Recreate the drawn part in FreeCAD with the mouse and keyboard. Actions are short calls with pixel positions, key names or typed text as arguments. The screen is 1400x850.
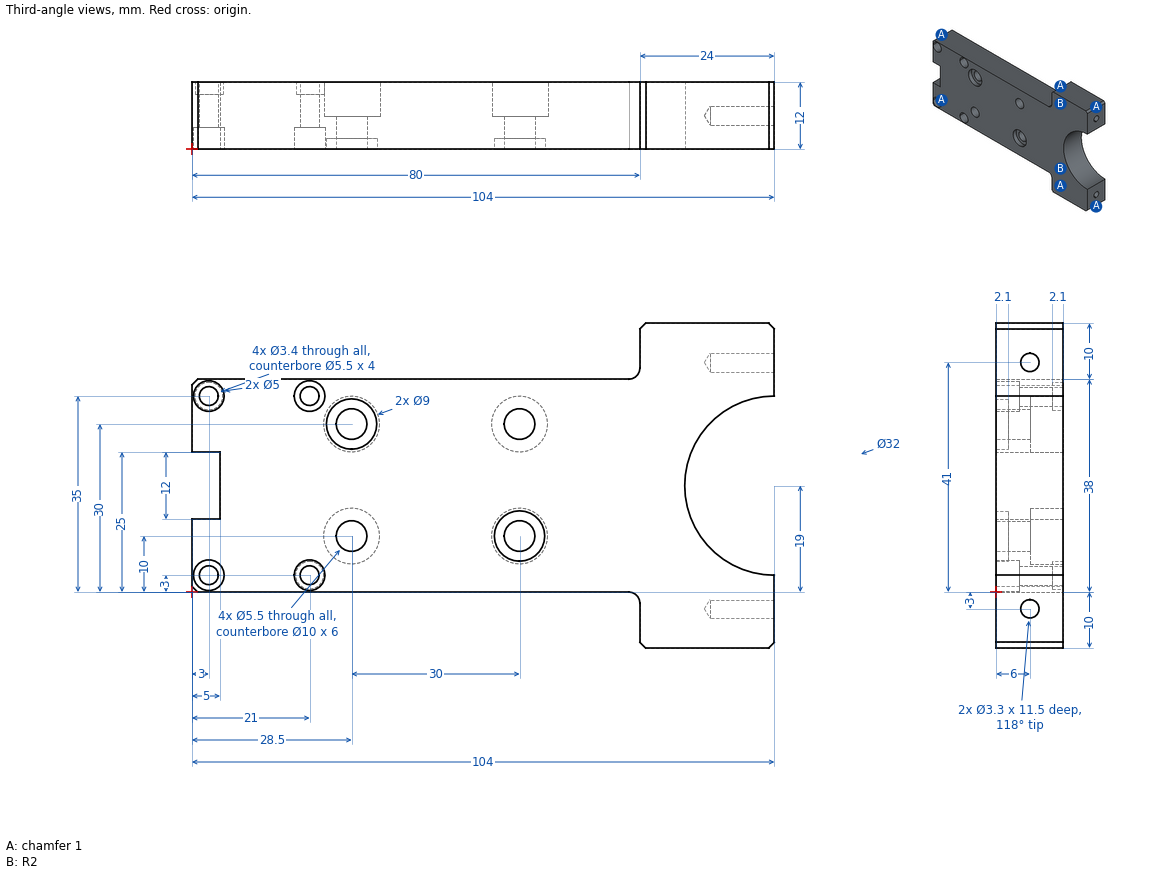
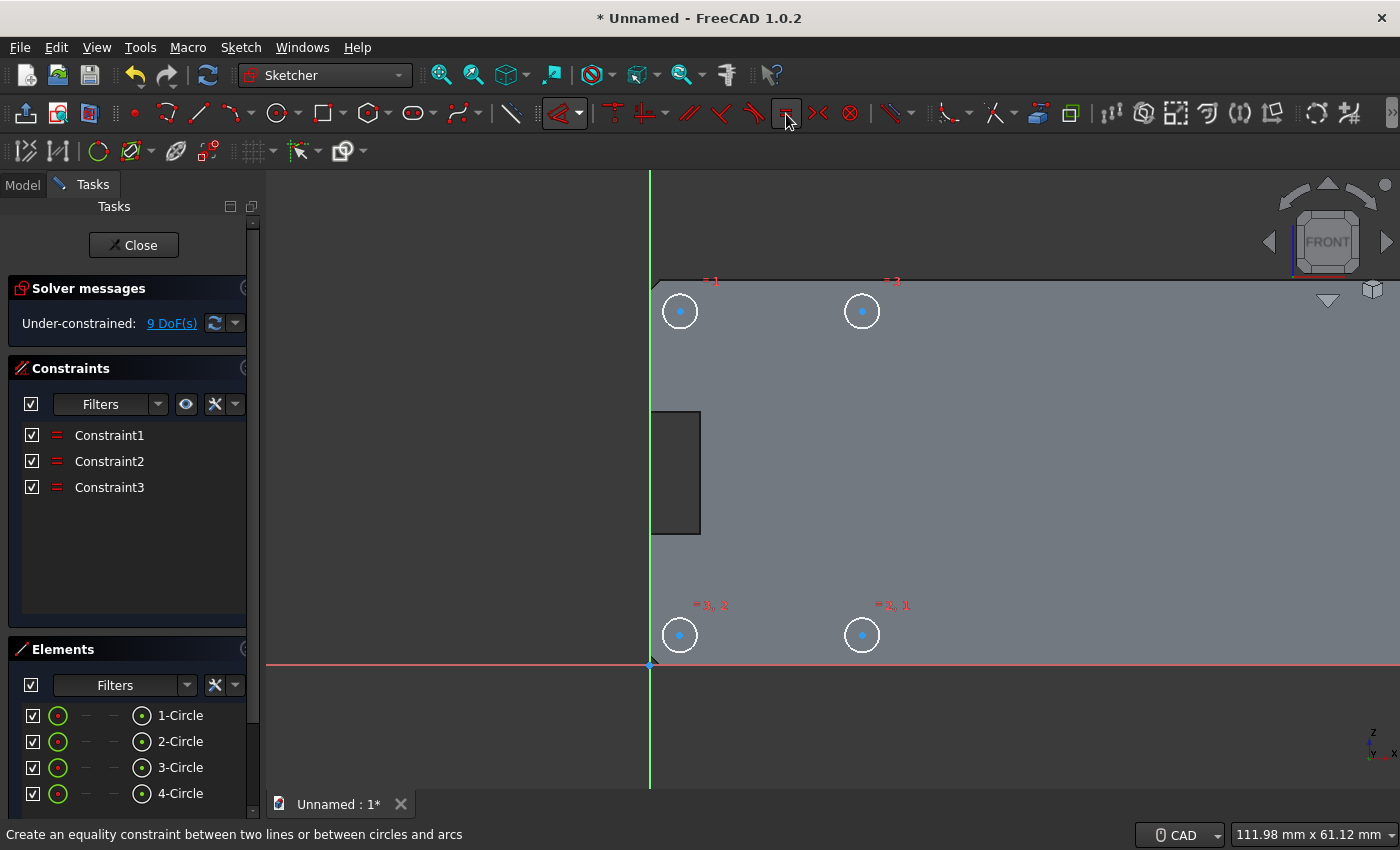
click(680, 311)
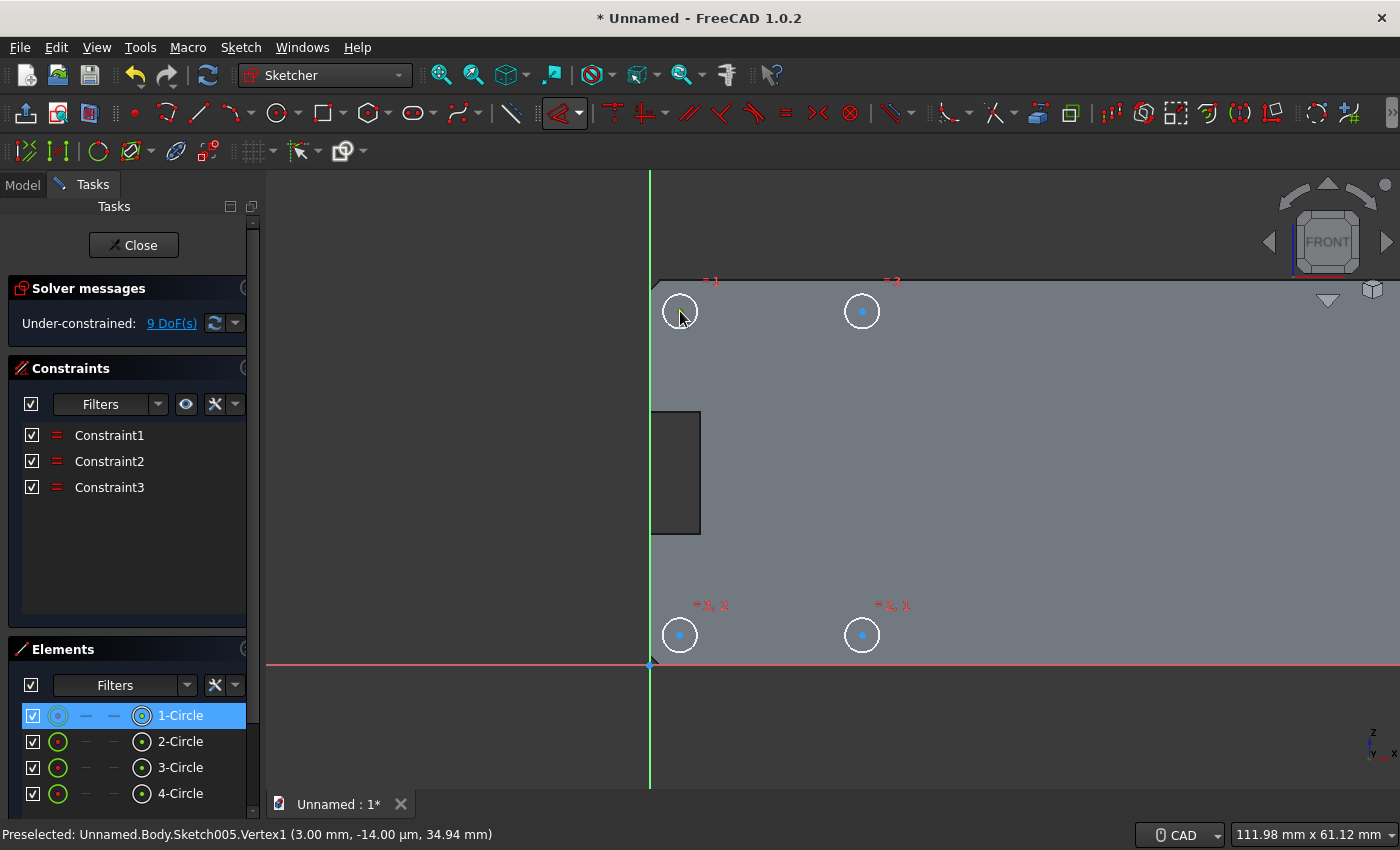
click(680, 635)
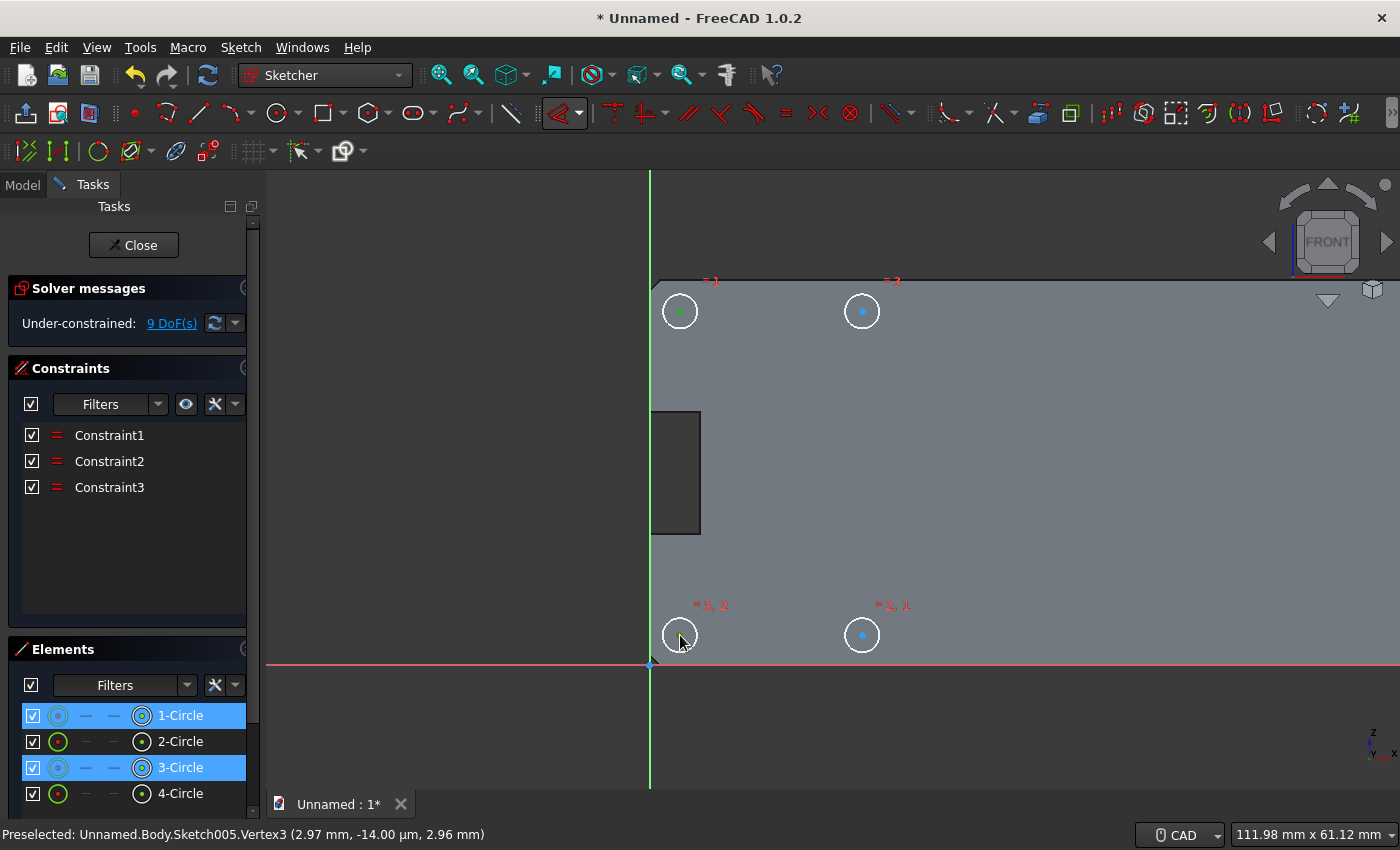
click(668, 114)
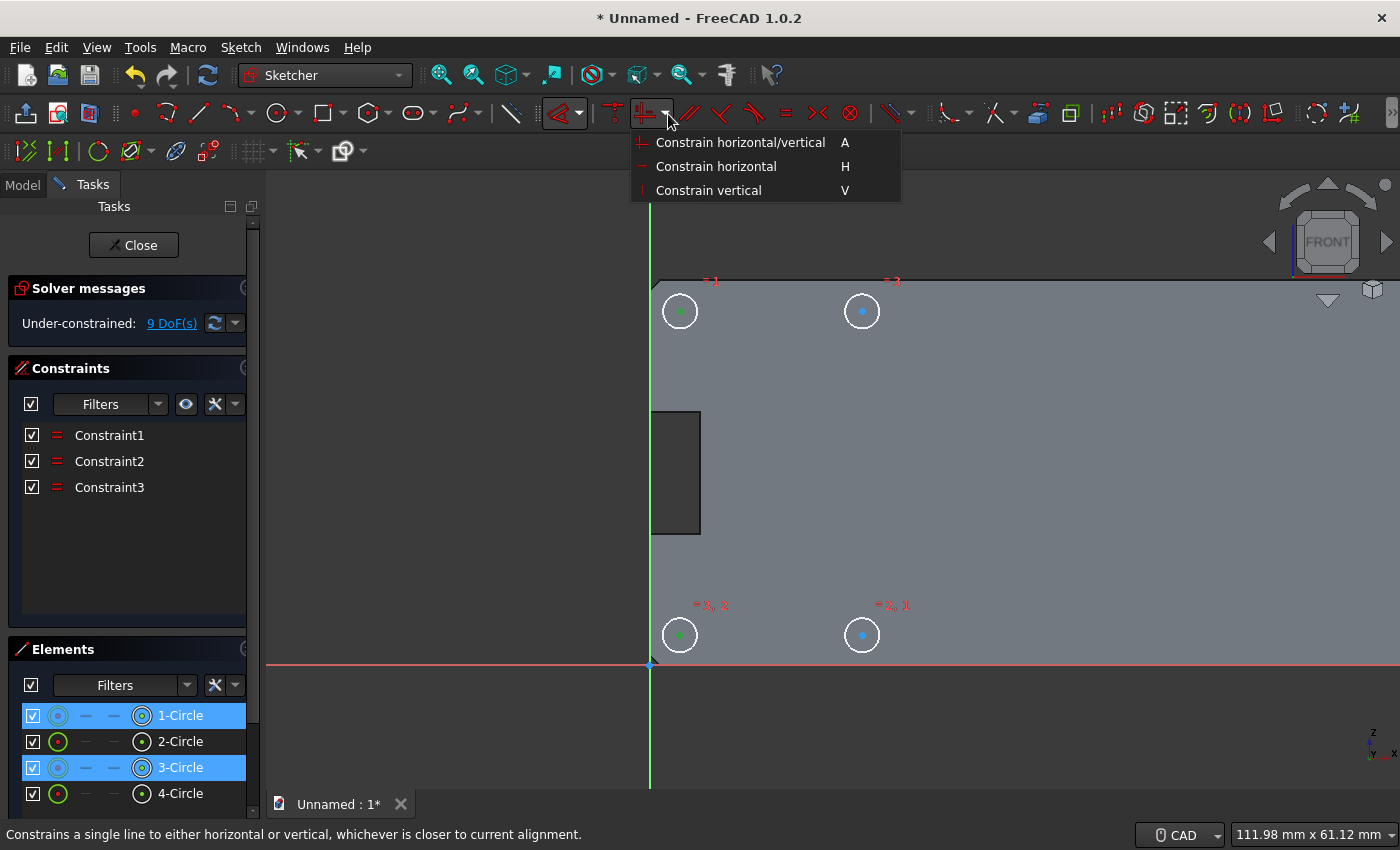
click(766, 190)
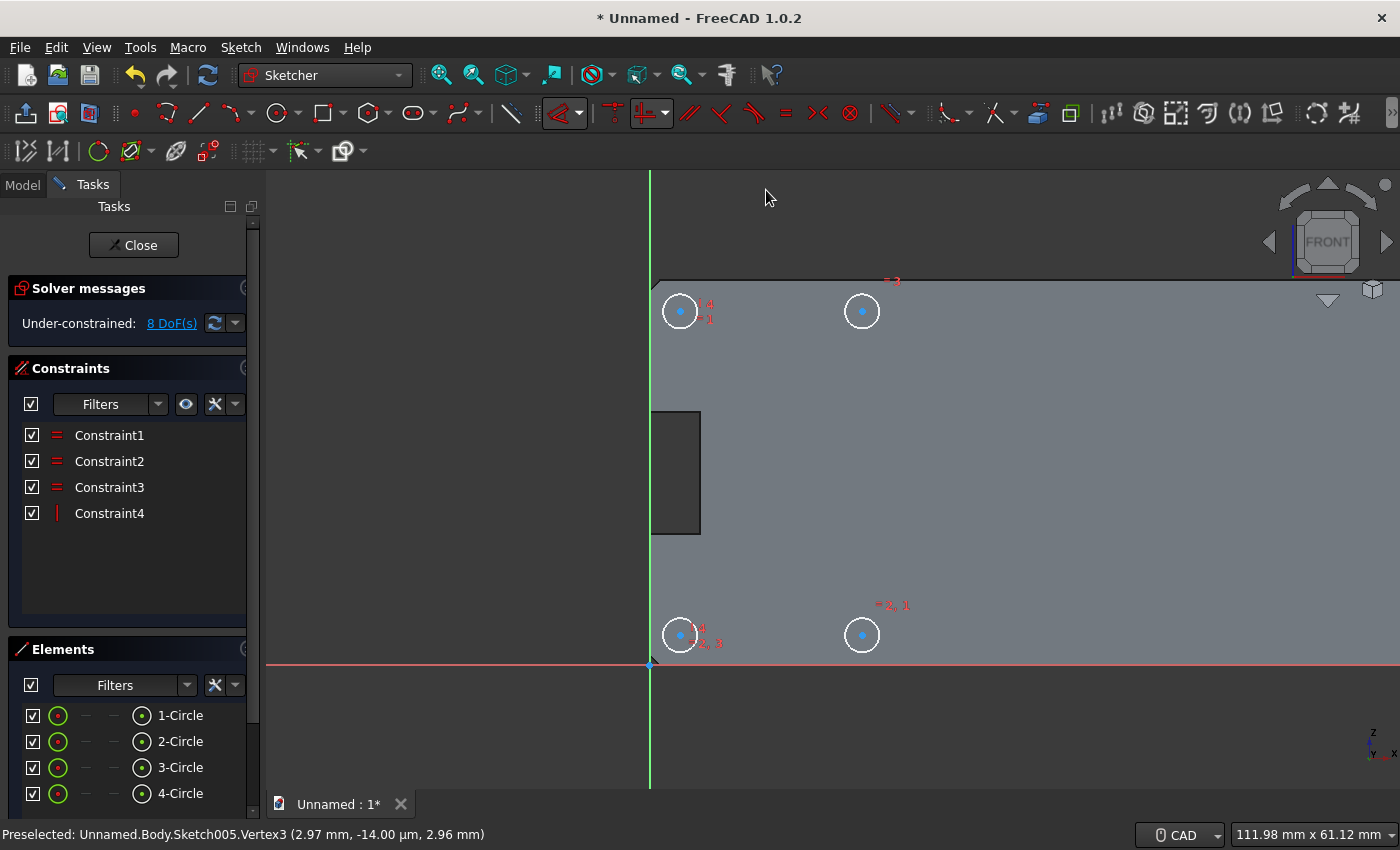
click(862, 635)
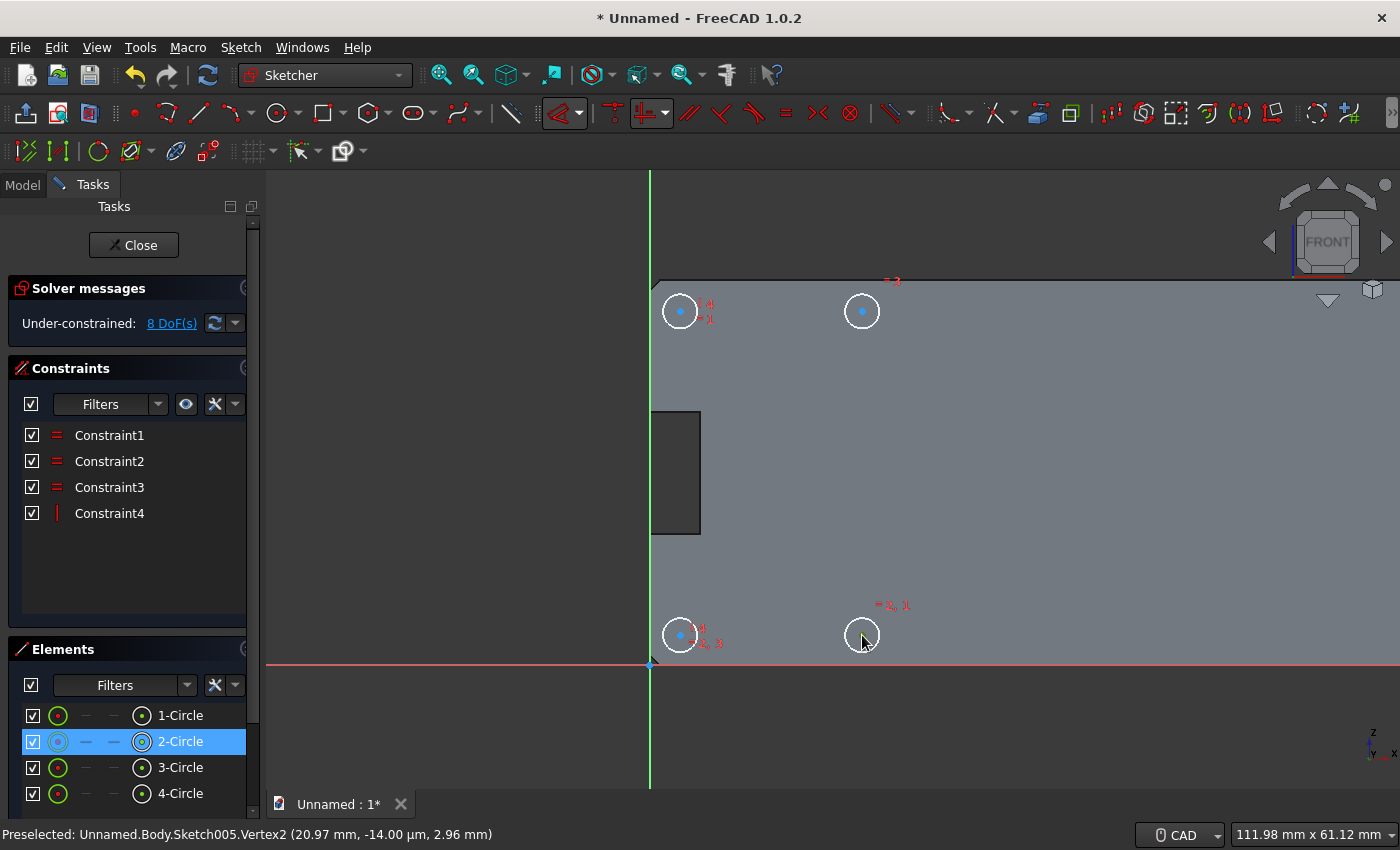
click(680, 635)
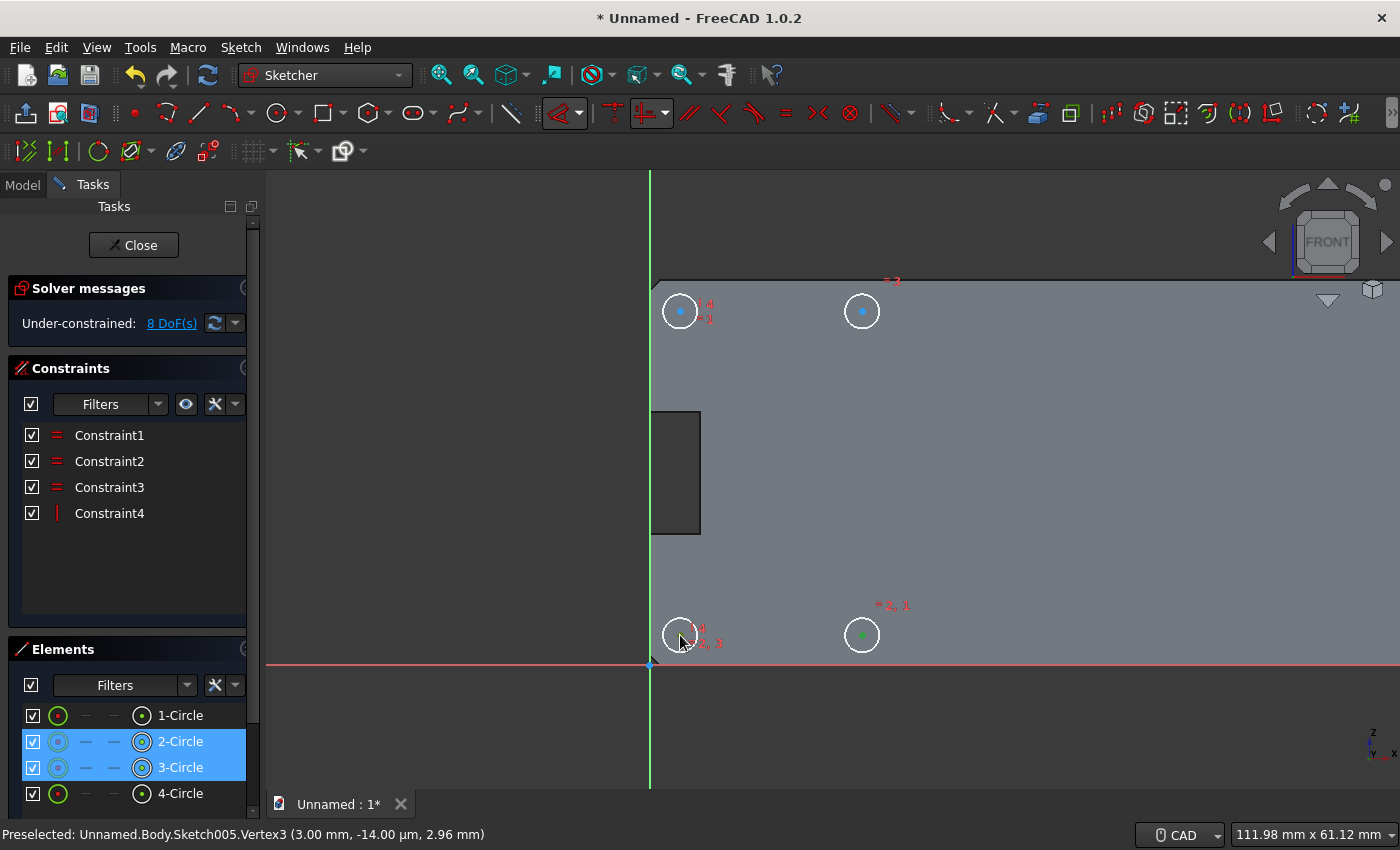
click(668, 114)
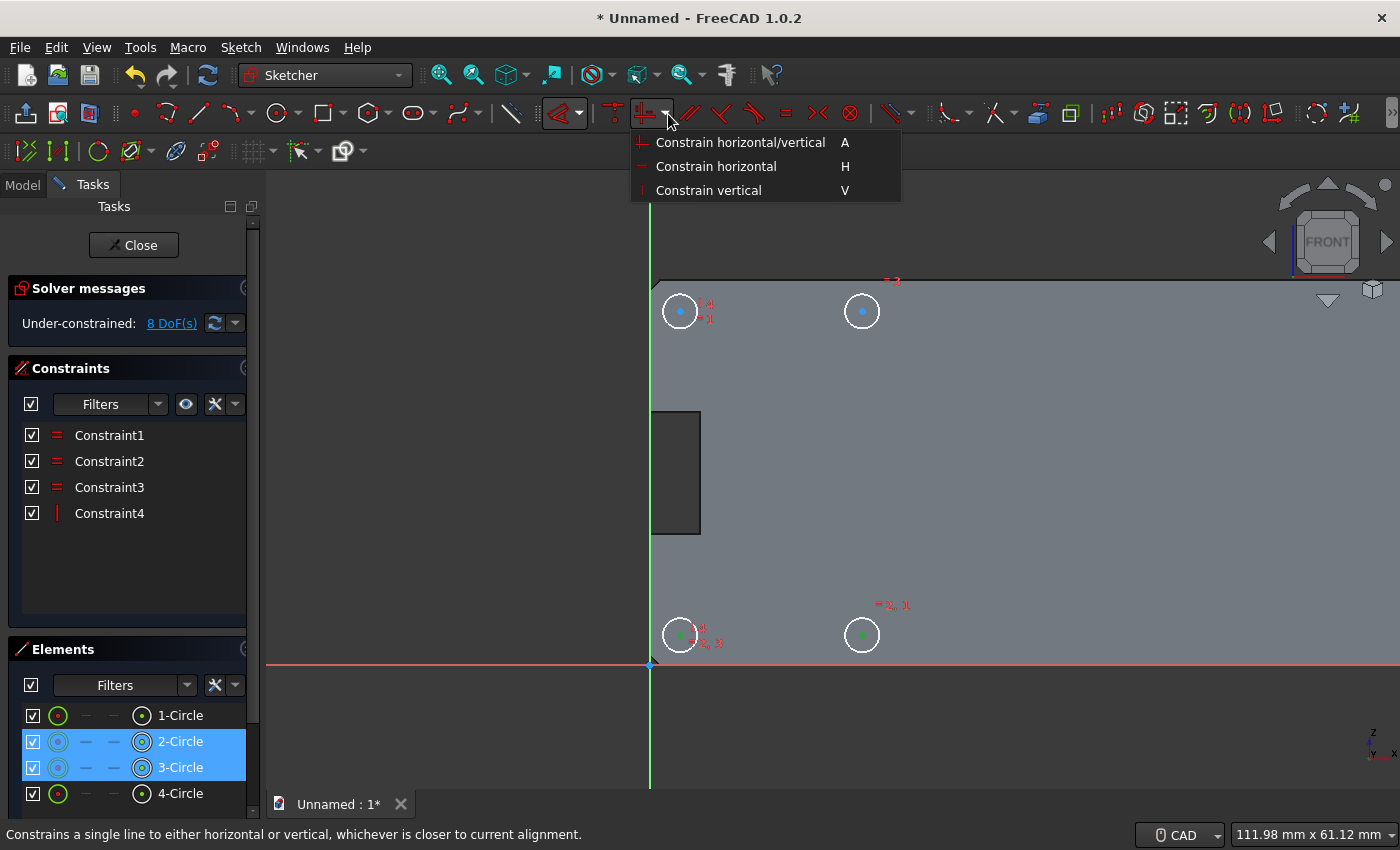
click(766, 166)